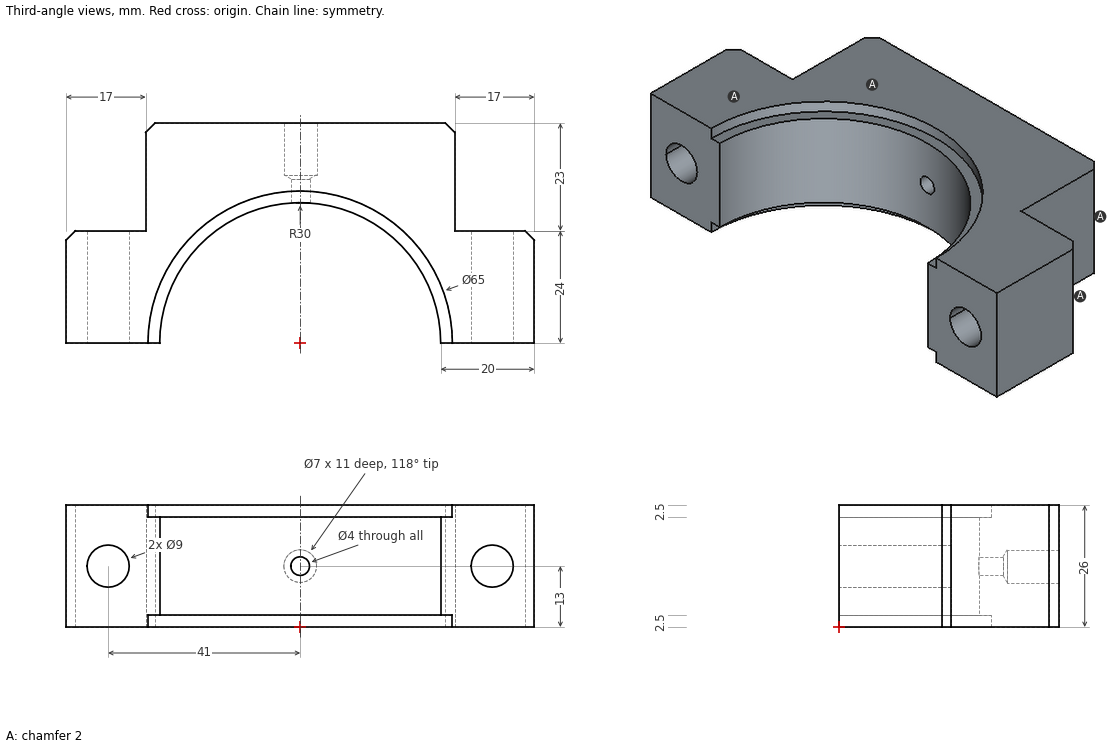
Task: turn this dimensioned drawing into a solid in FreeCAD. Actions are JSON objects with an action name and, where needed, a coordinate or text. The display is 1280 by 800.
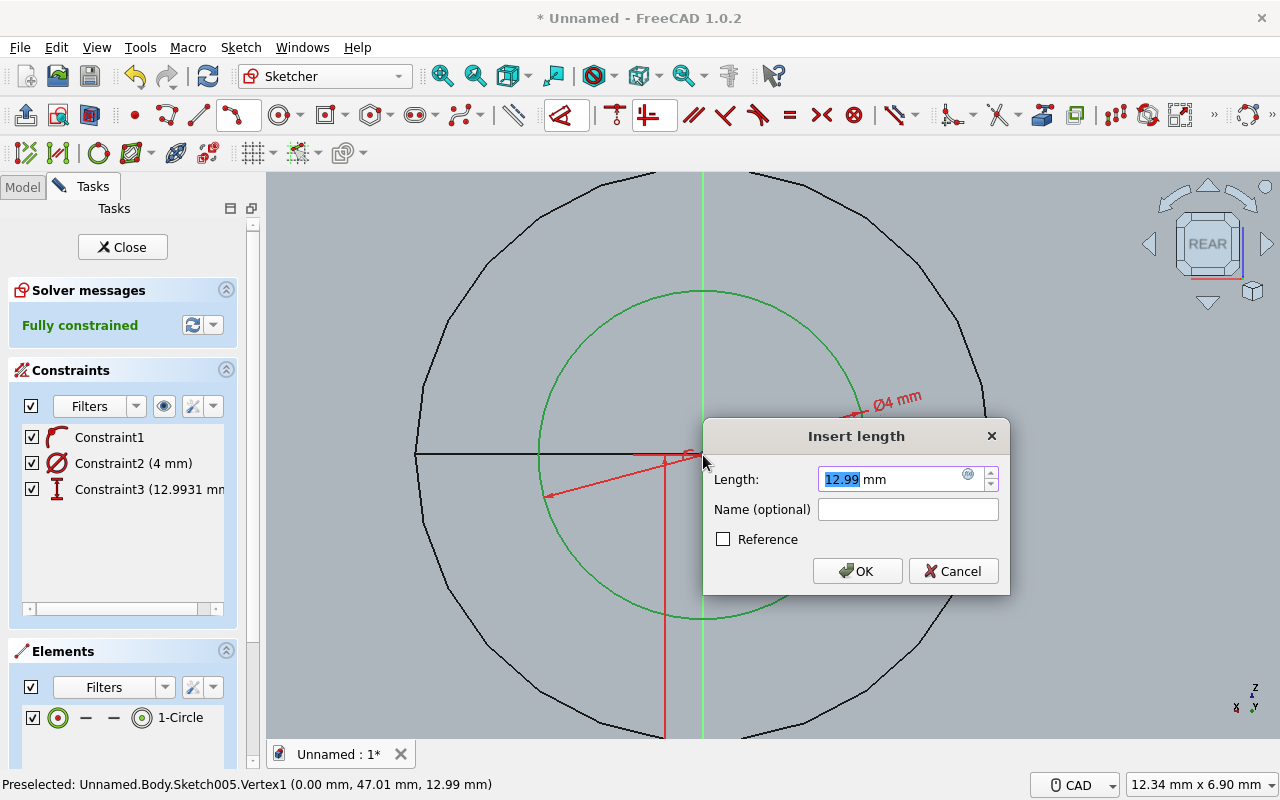
{"action": "type", "text": "13"}
{"action": "key", "text": "Return"}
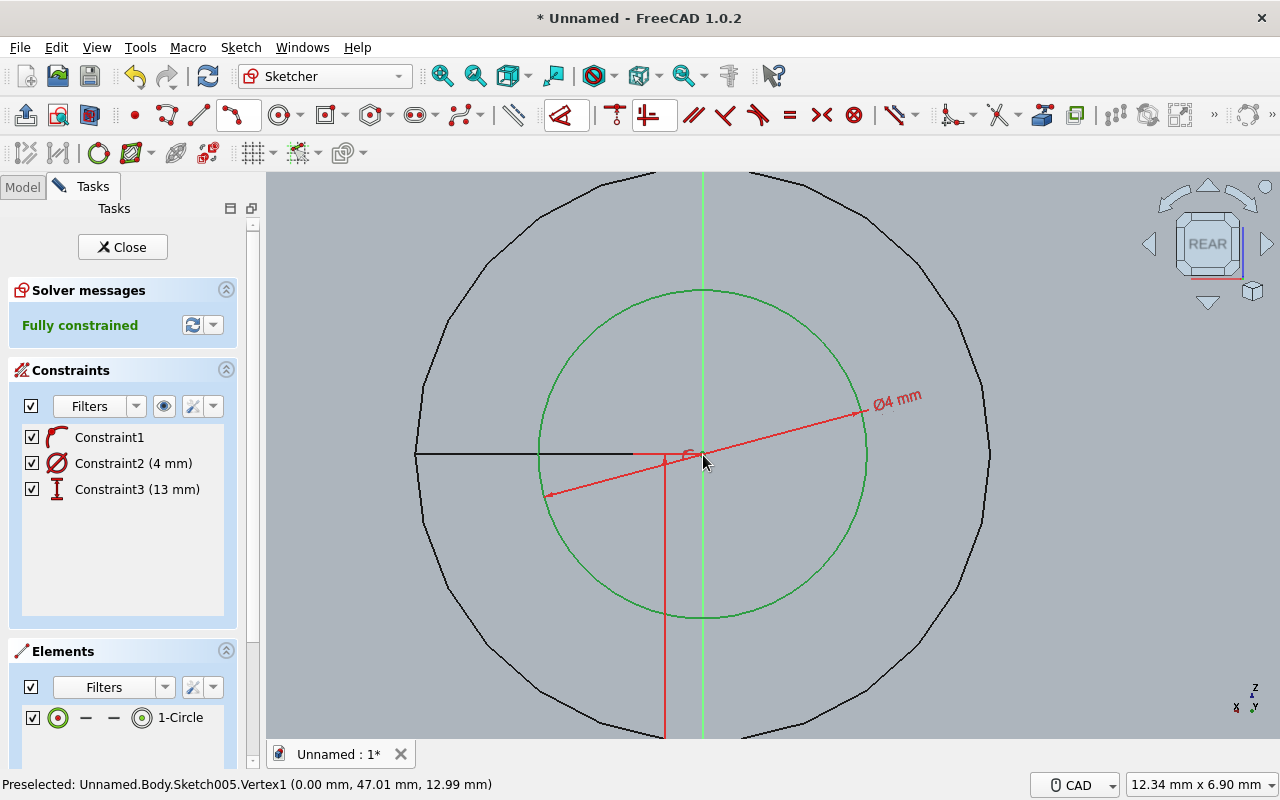
{"action": "left_click", "coordinate": [123, 247]}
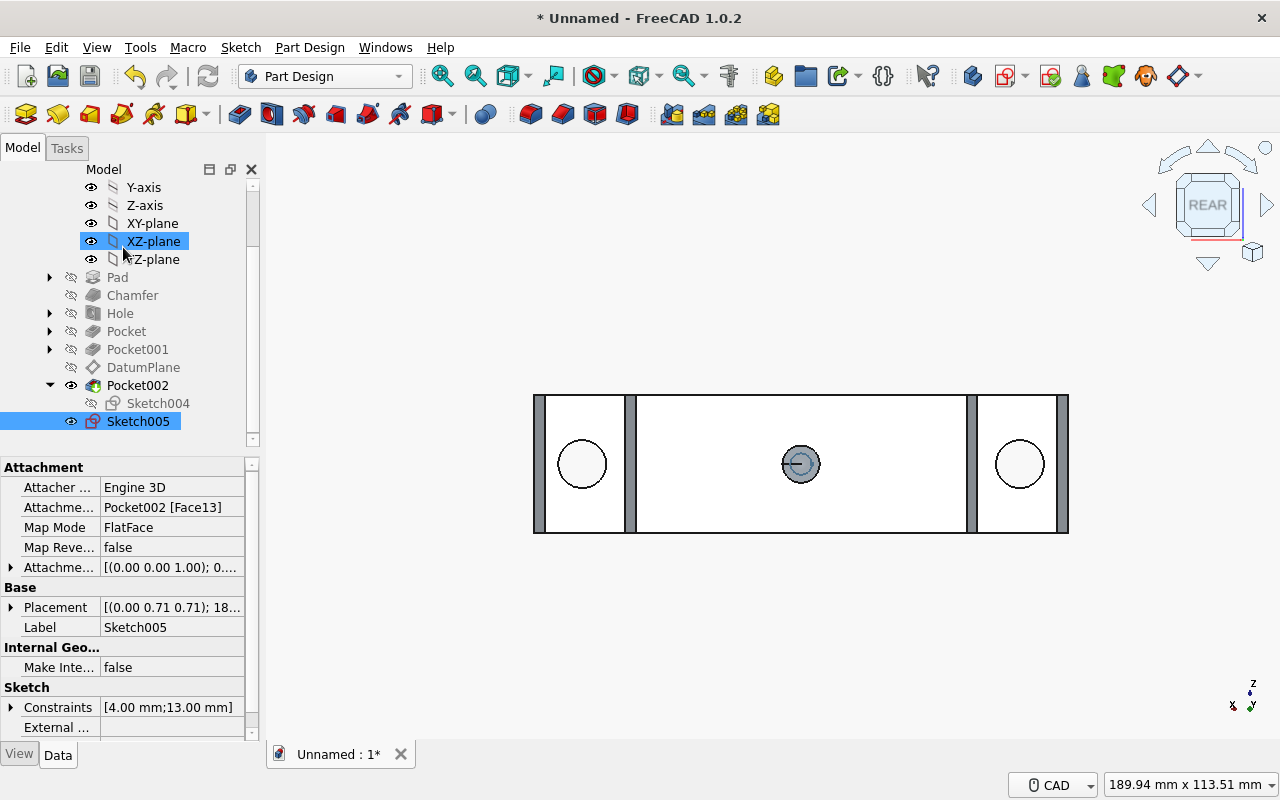
{"action": "left_click", "coordinate": [272, 114]}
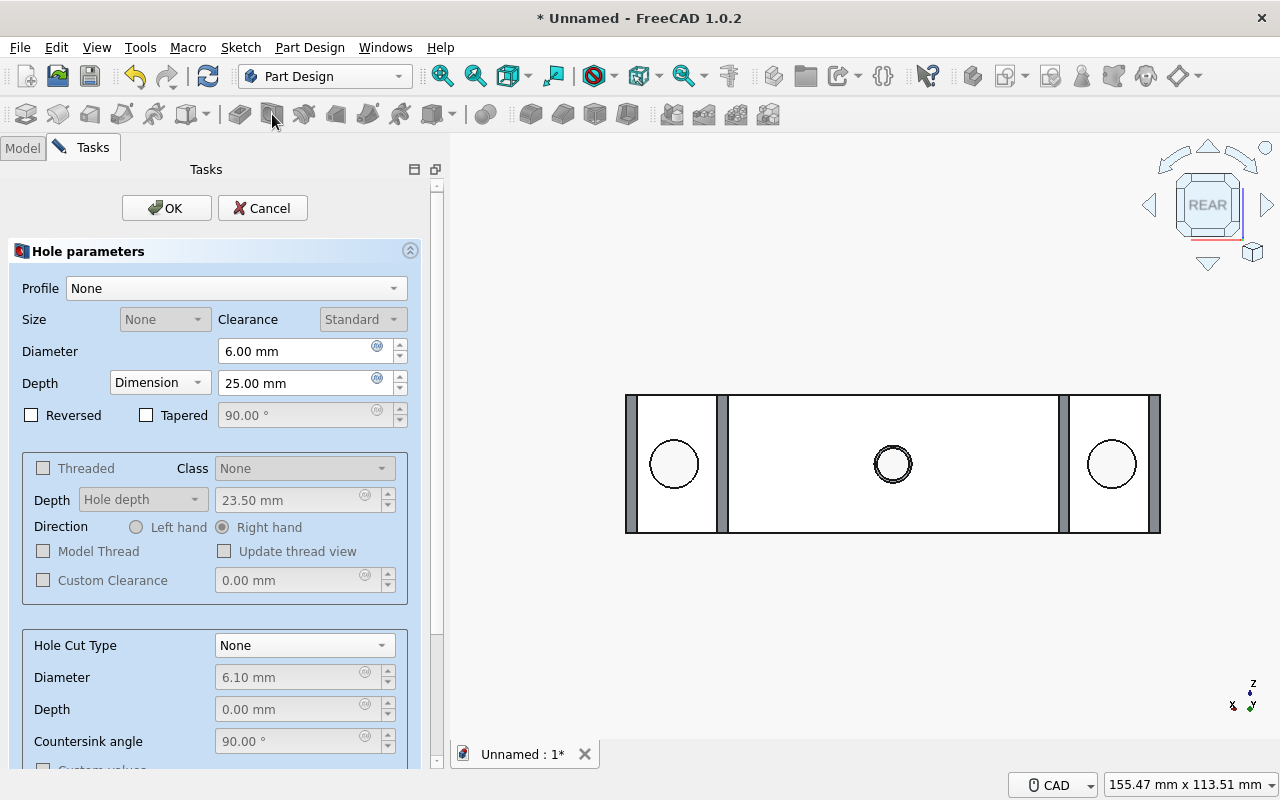
{"action": "triple_click", "coordinate": [305, 351]}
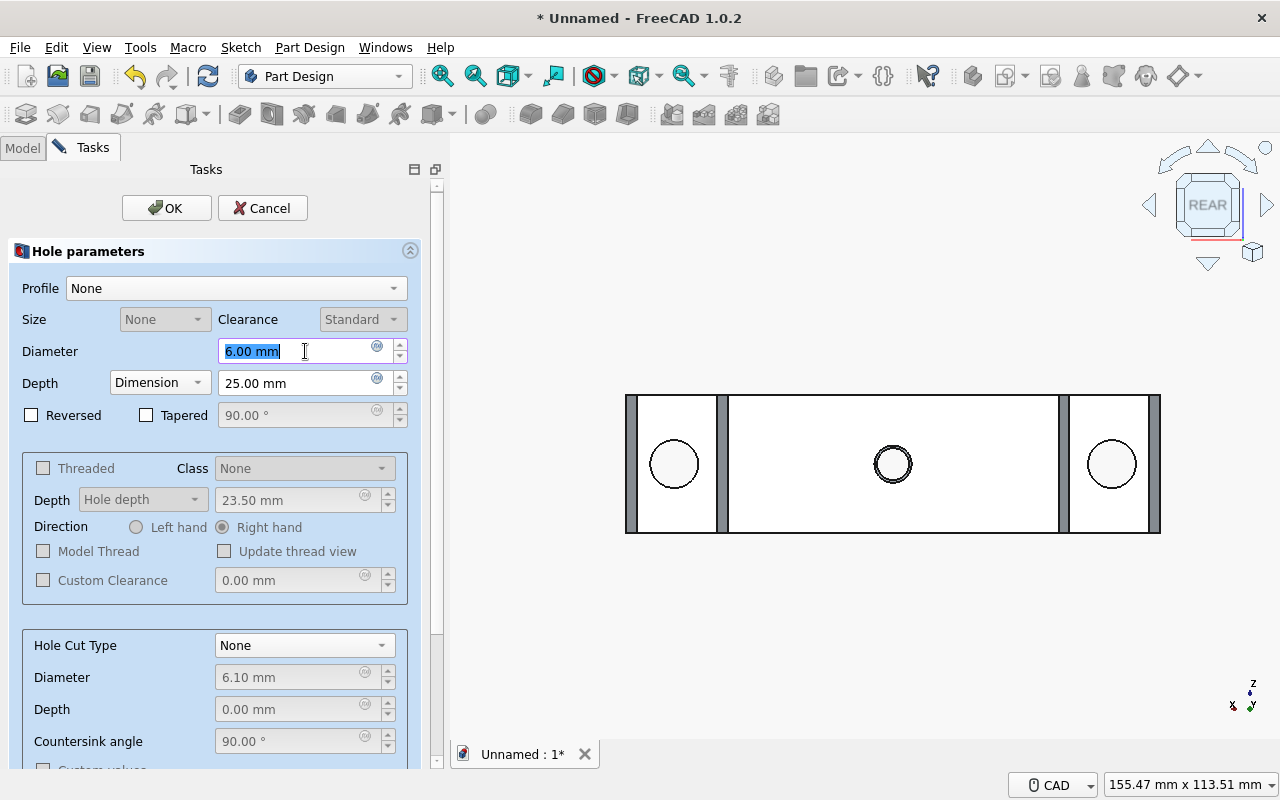
{"action": "type", "text": "4"}
{"action": "key", "text": "Tab"}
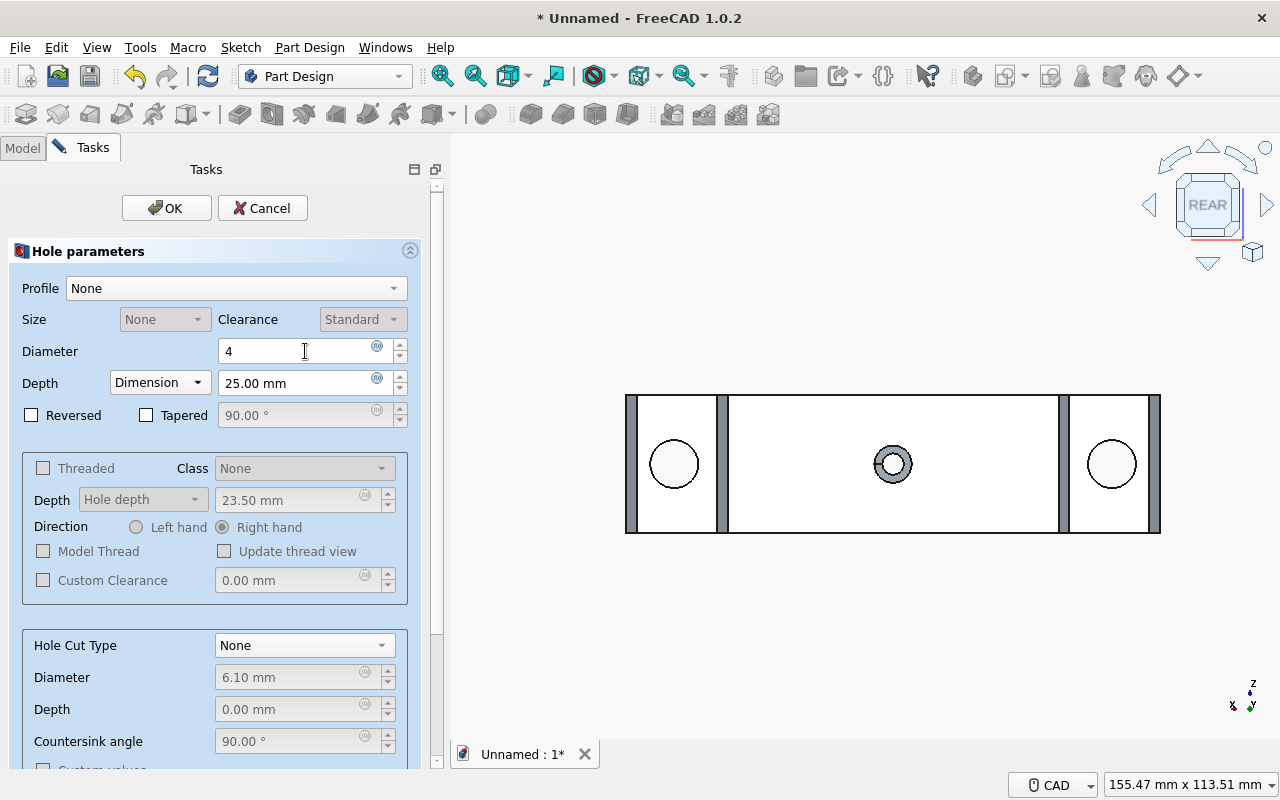
{"action": "left_click", "coordinate": [161, 382]}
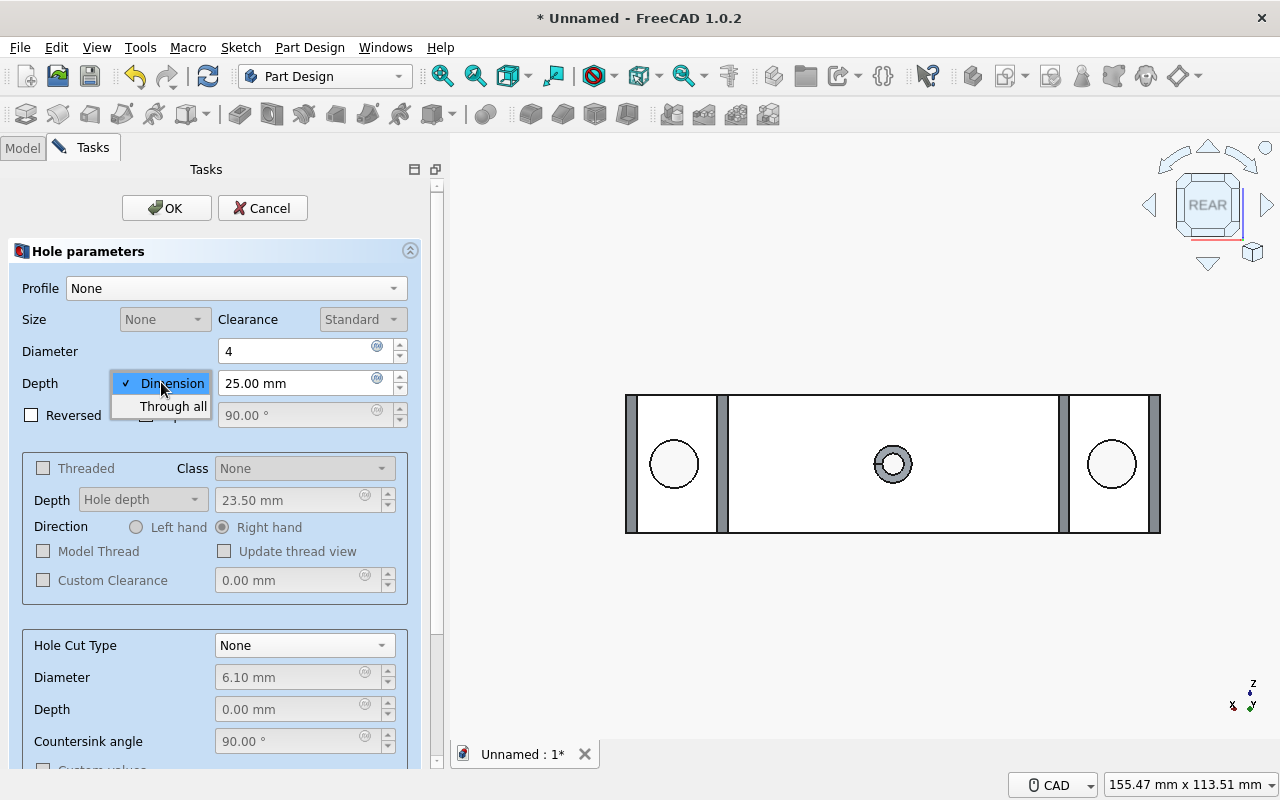
{"action": "left_click", "coordinate": [160, 406]}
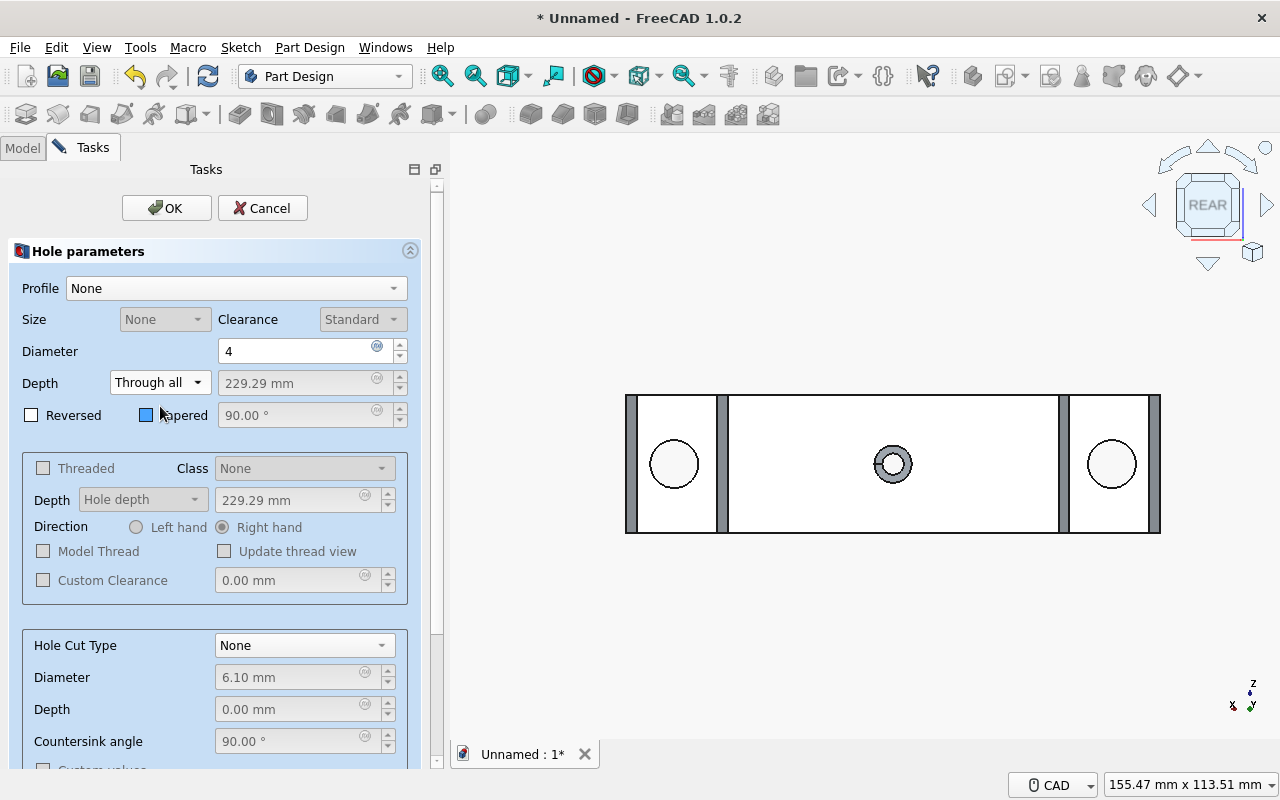
{"action": "left_click", "coordinate": [167, 208]}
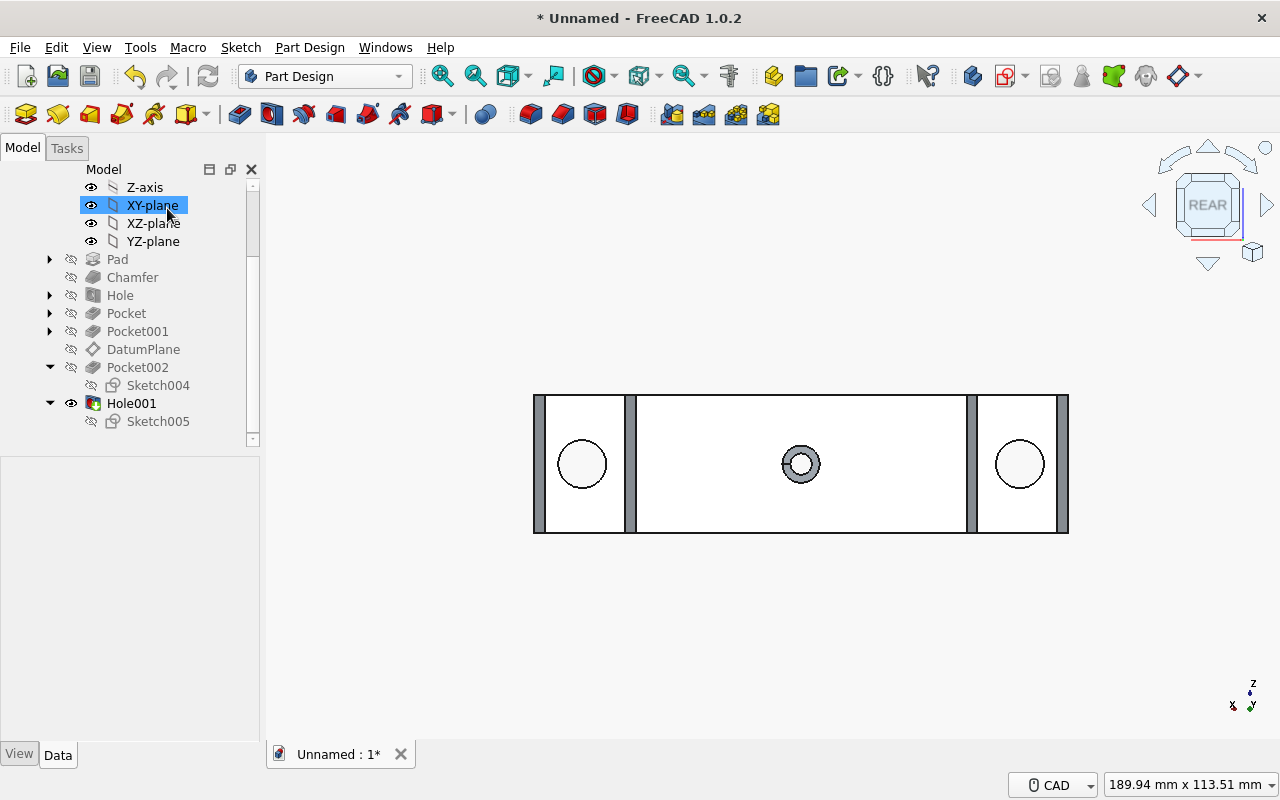
{"action": "key", "text": "0"}